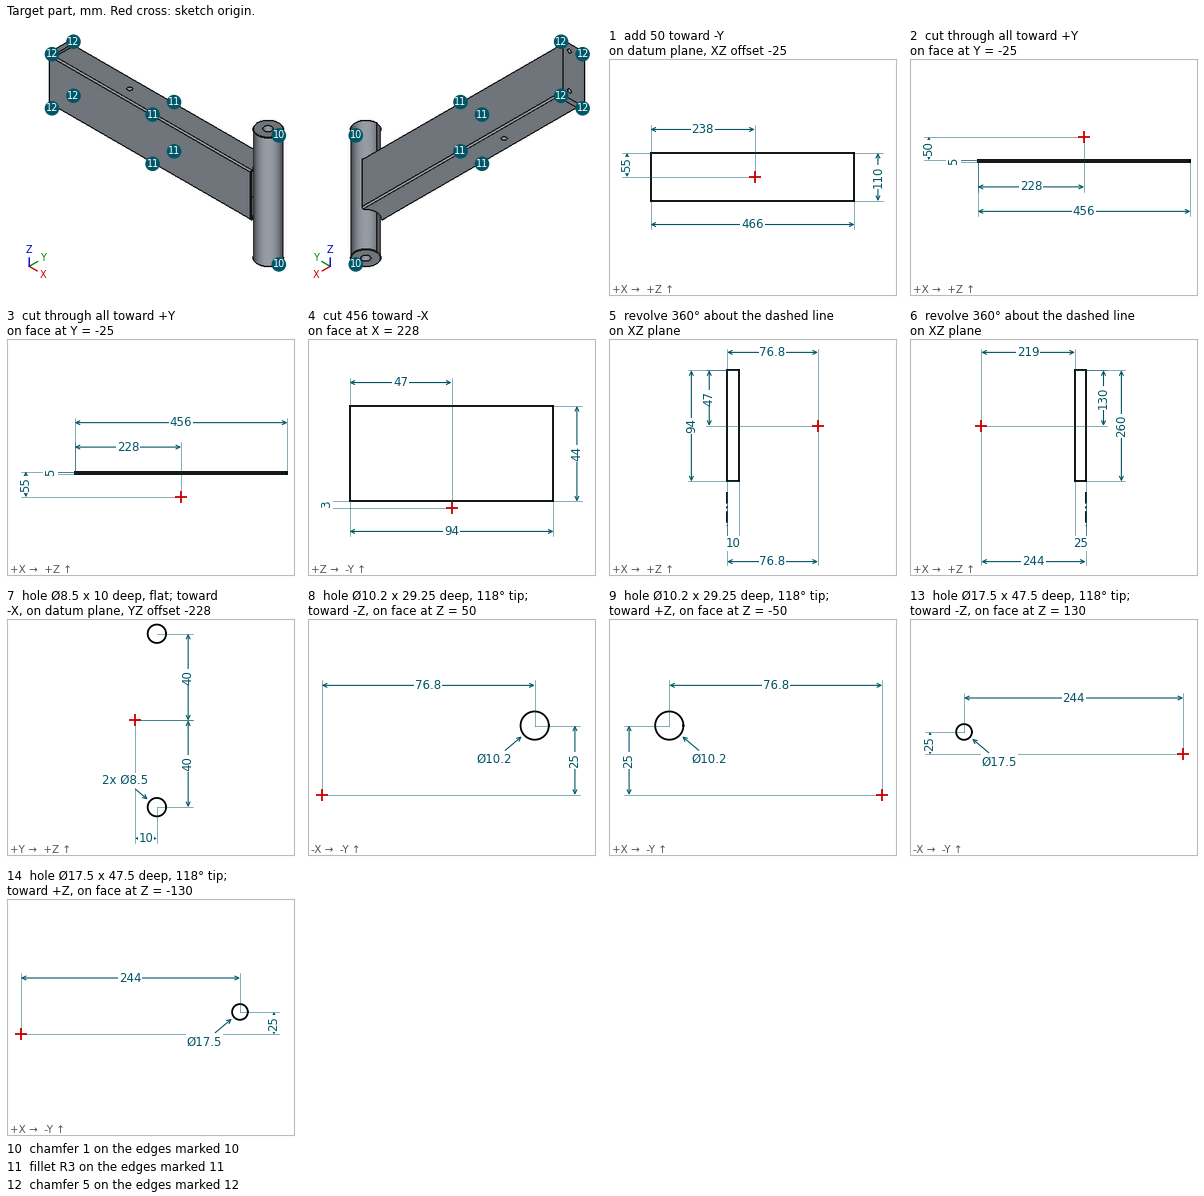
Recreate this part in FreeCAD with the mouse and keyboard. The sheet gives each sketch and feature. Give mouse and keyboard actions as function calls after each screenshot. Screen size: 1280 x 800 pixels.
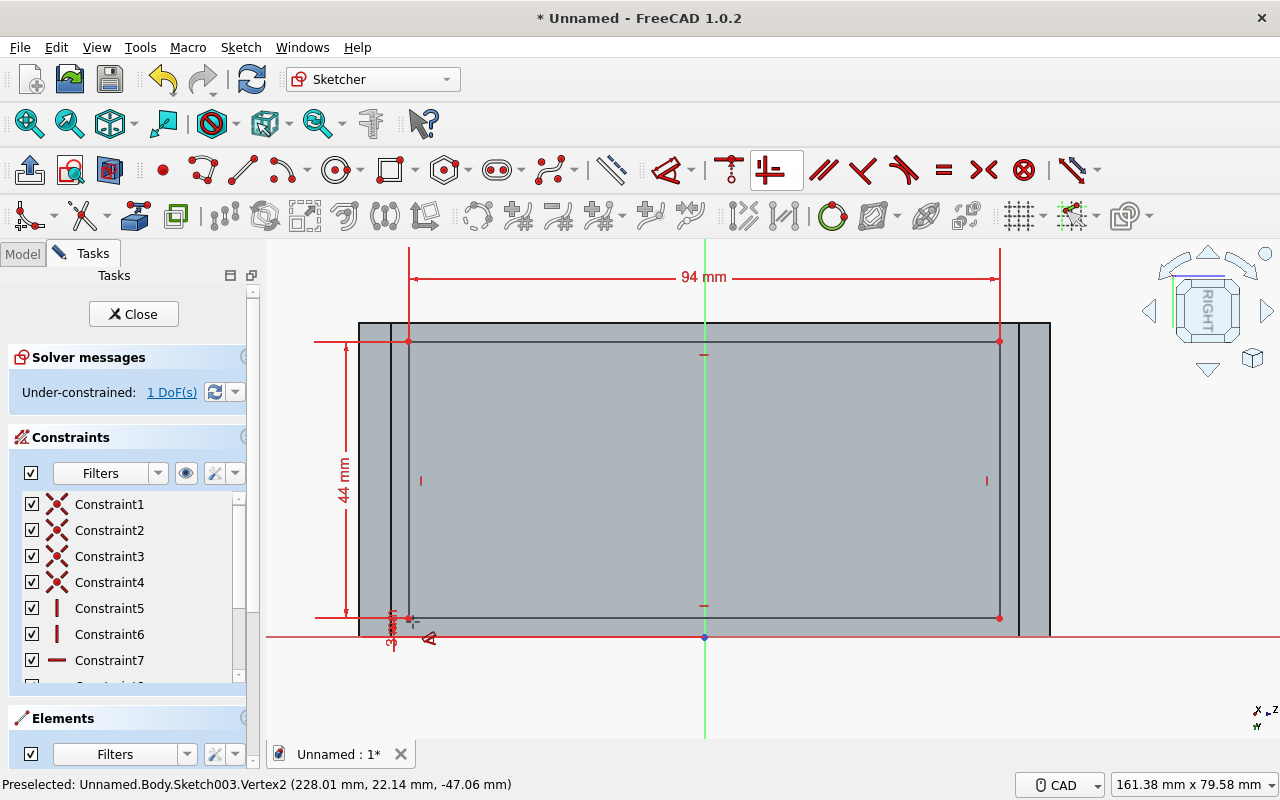
click(409, 342)
click(557, 671)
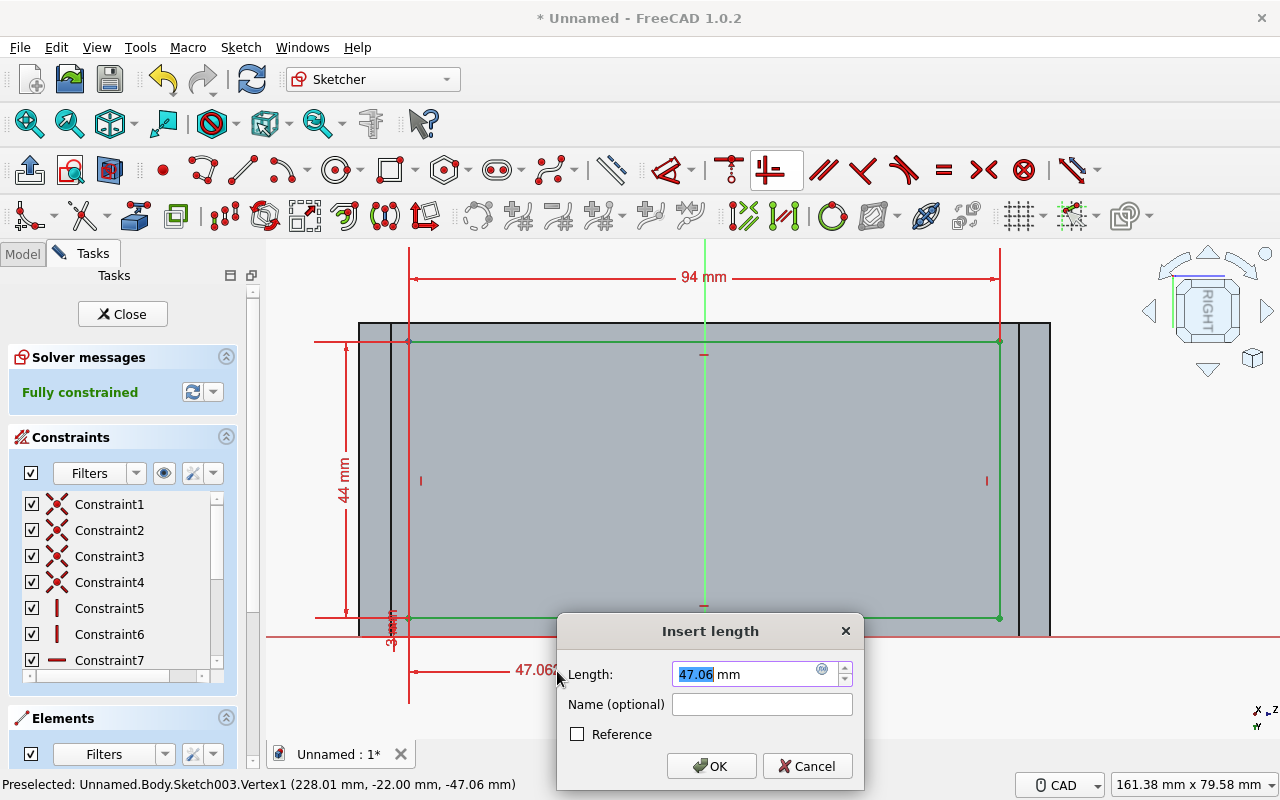
text(47)
key(Return)
key(Escape)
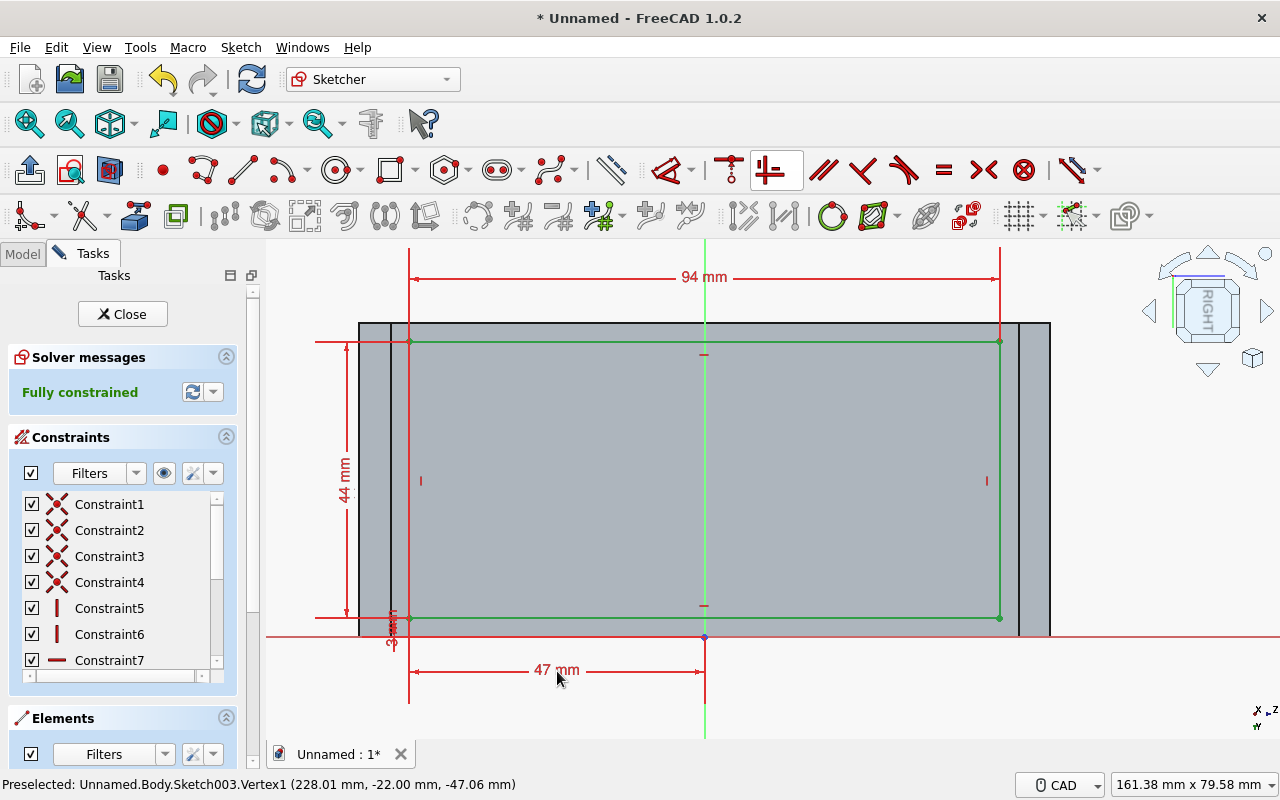
click(123, 314)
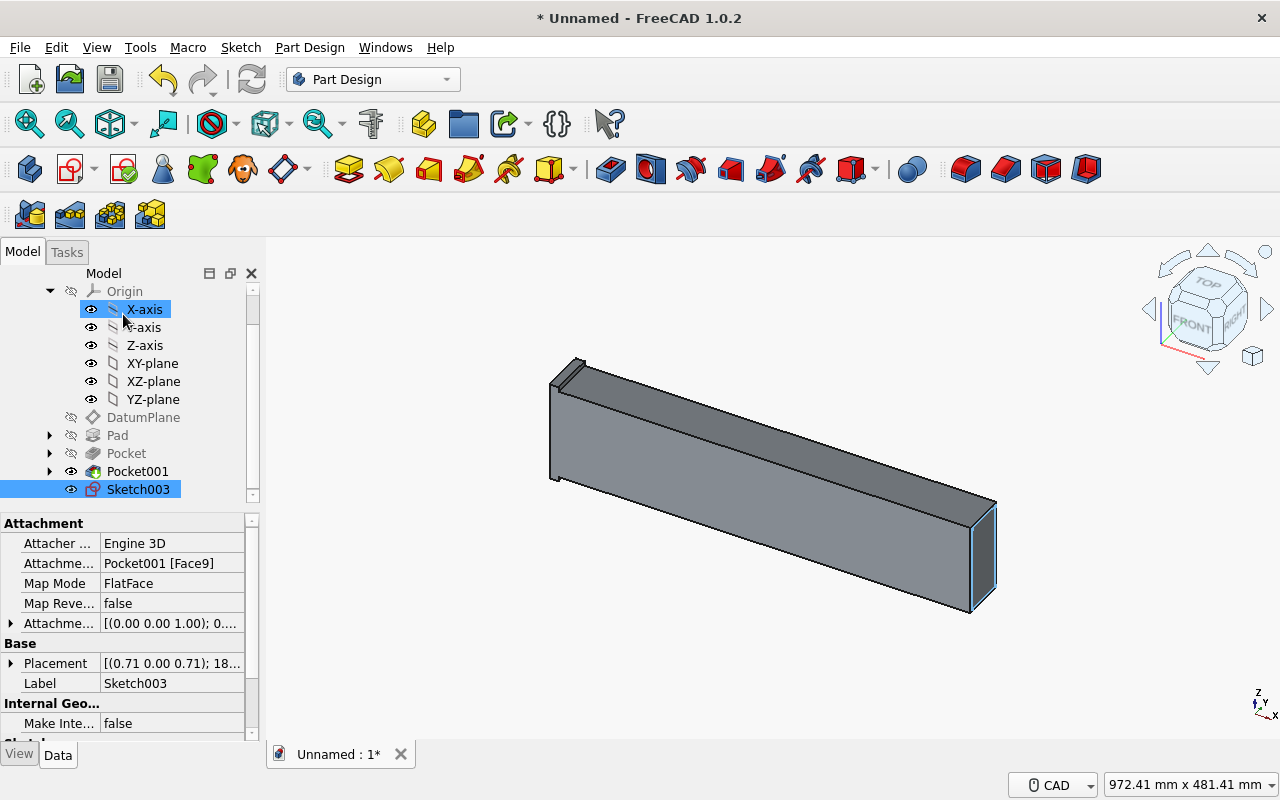
click(612, 170)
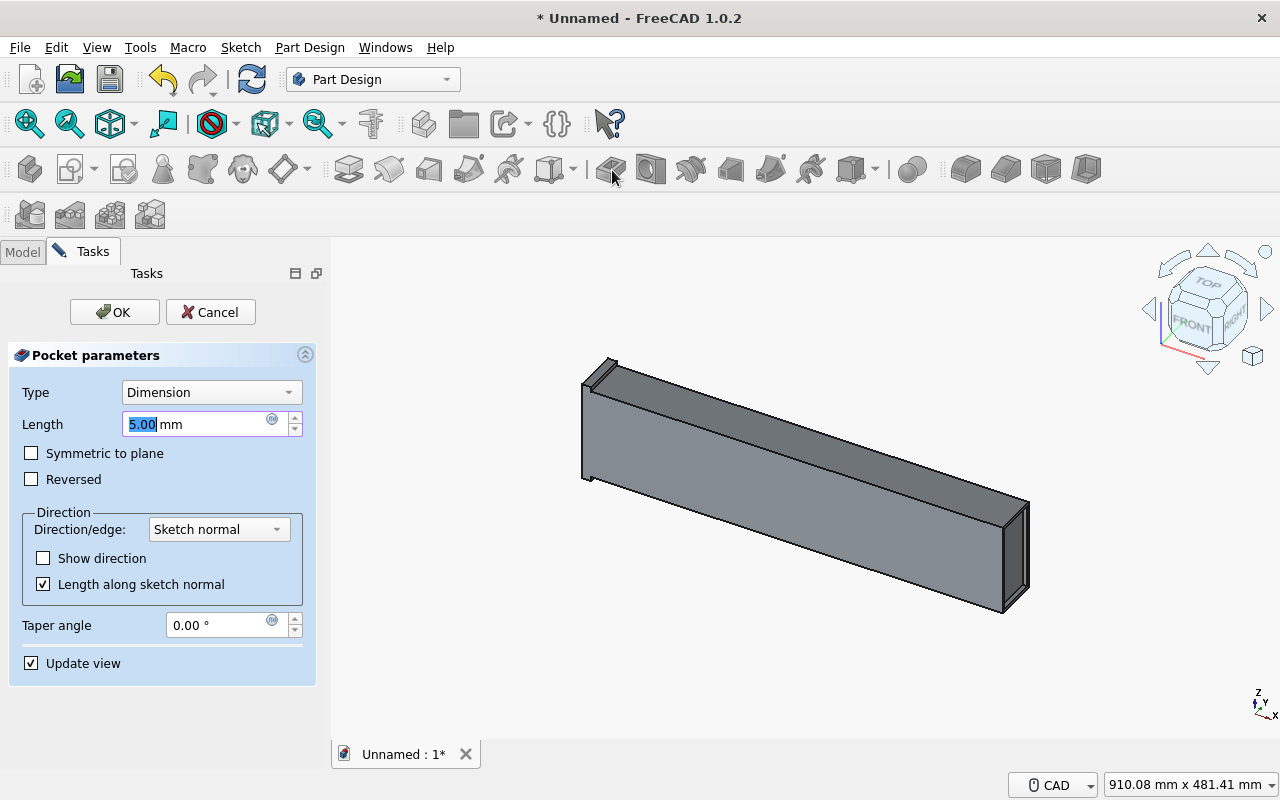
text(456)
key(Tab)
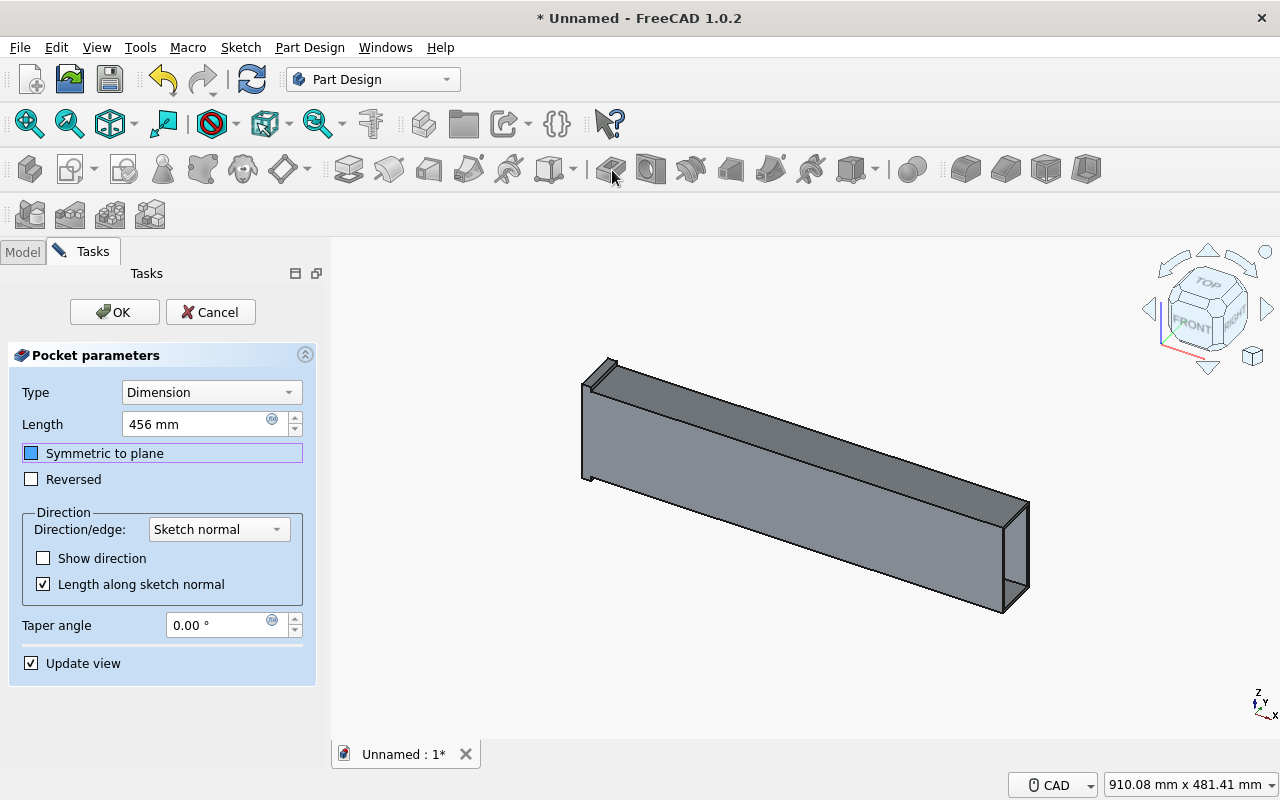
click(115, 312)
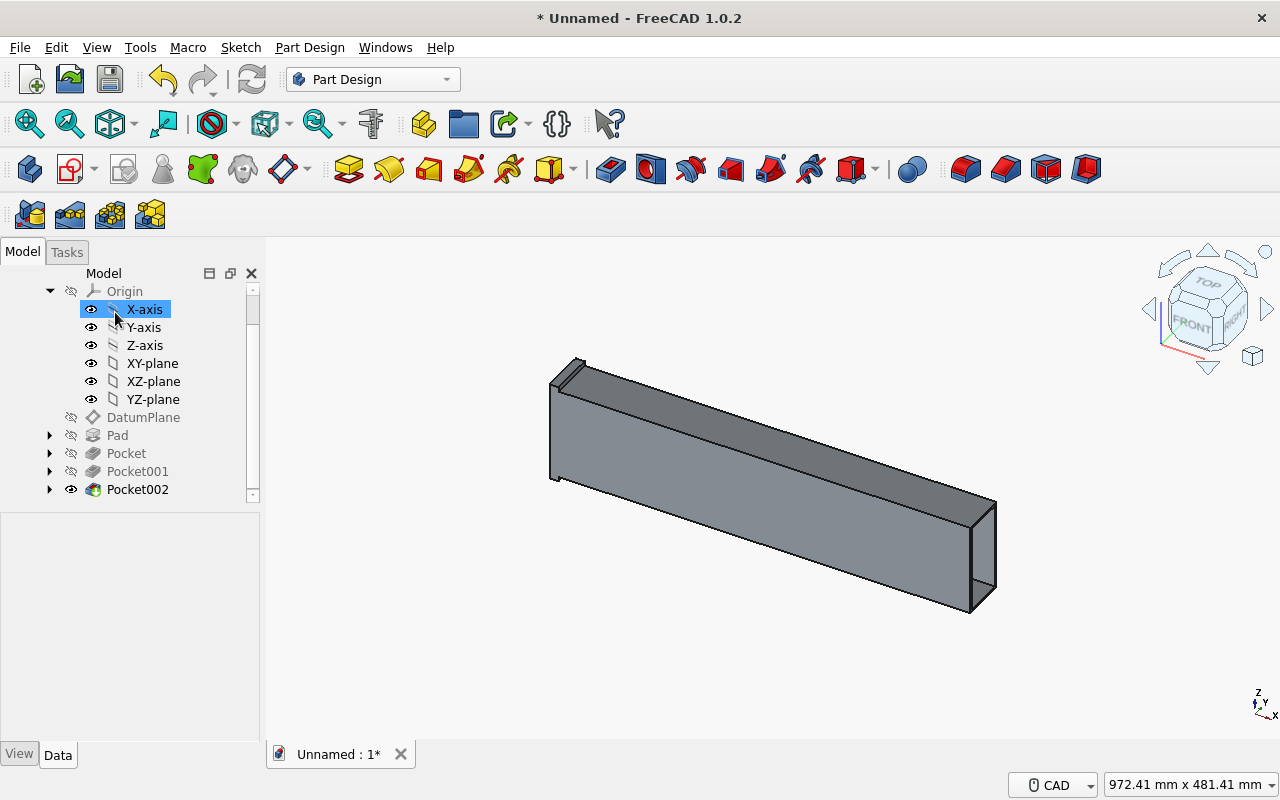
click(70, 170)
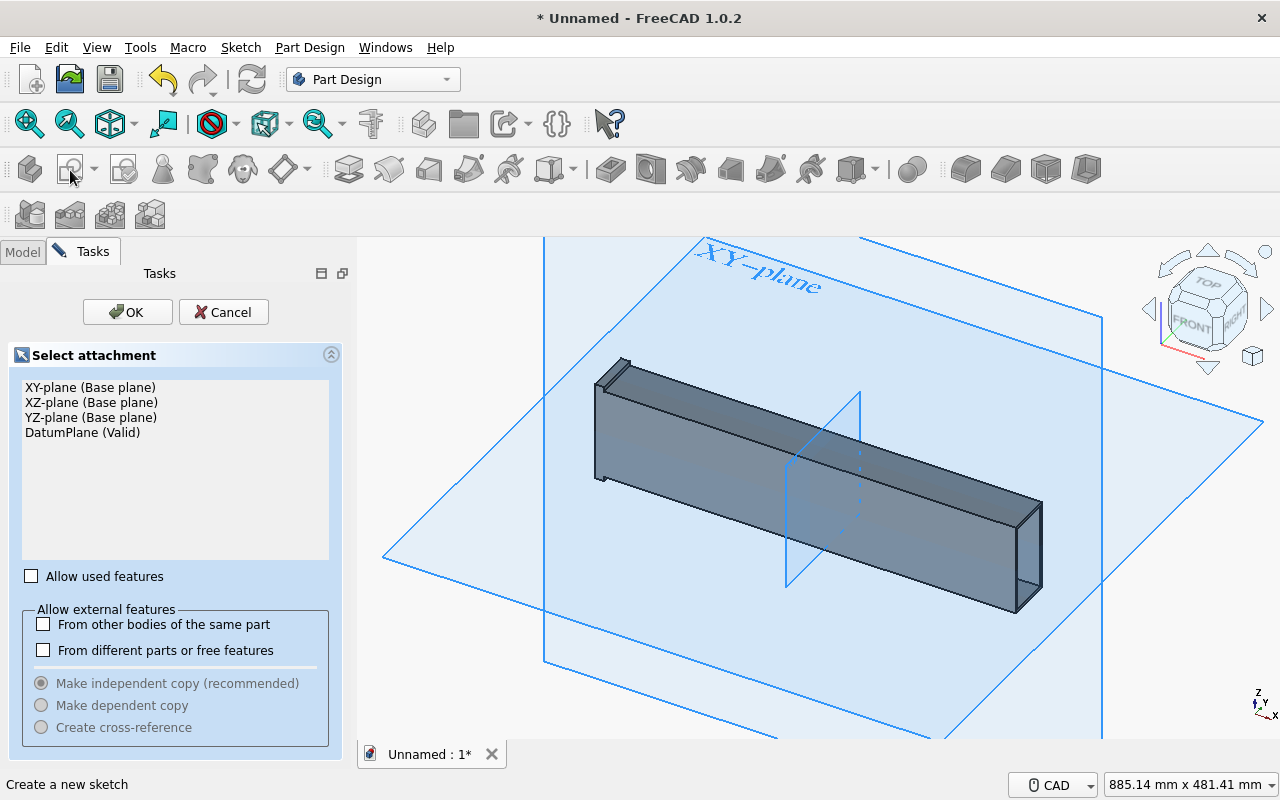
click(82, 402)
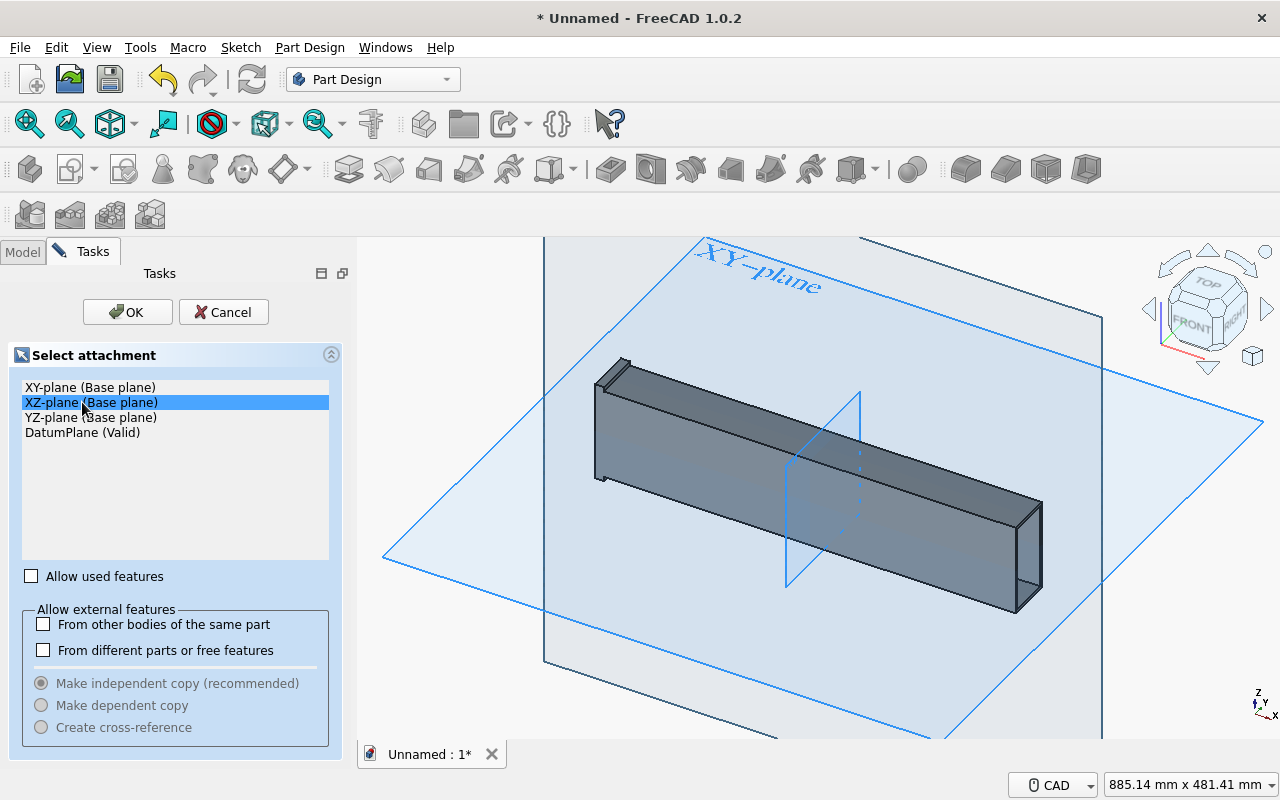
click(128, 312)